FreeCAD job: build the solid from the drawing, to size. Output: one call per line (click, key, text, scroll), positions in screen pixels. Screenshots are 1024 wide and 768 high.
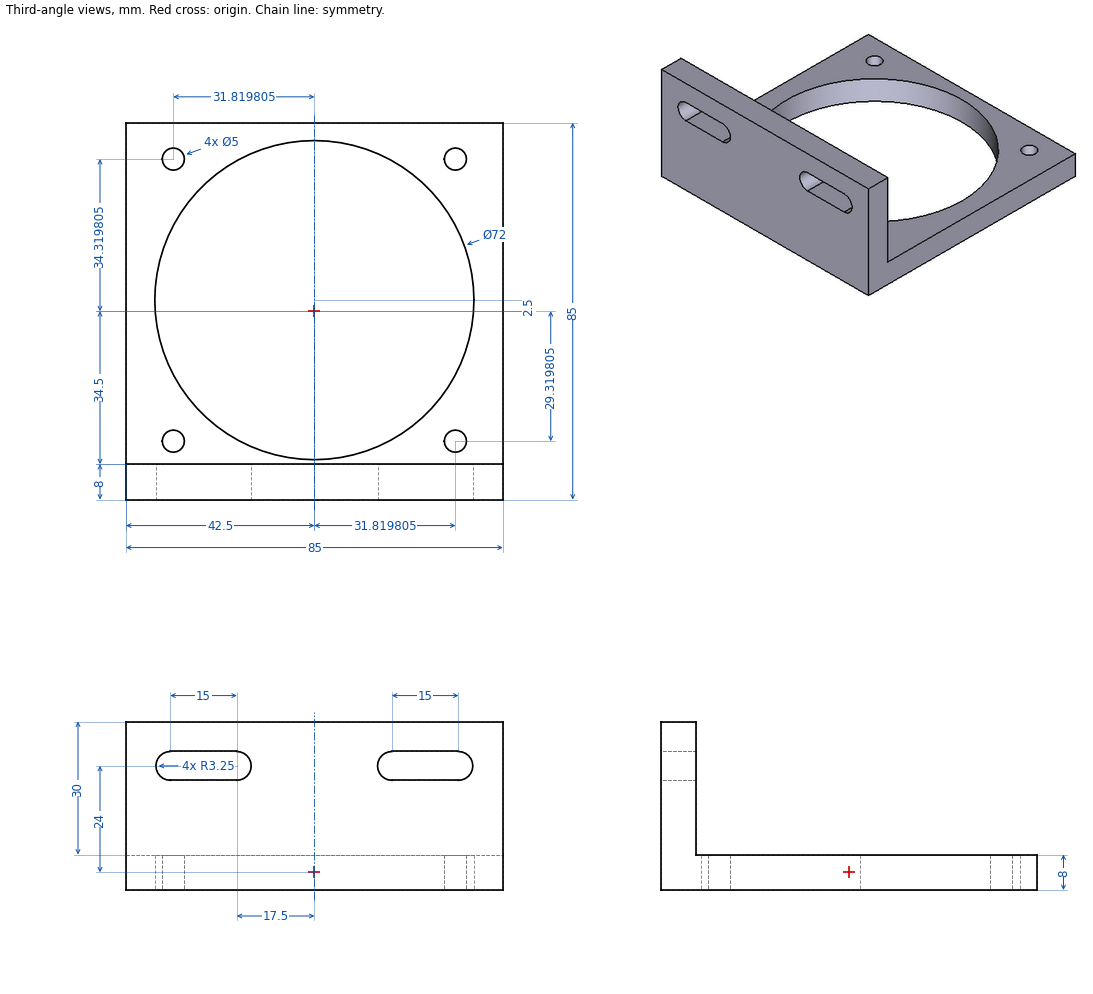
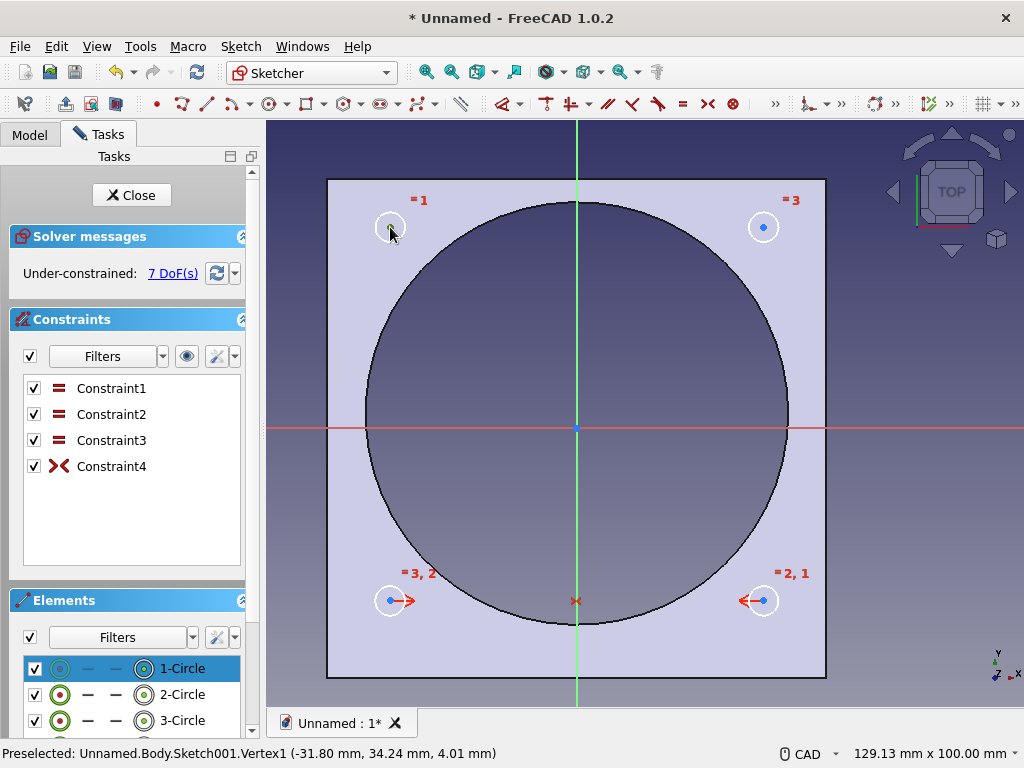
click(764, 227)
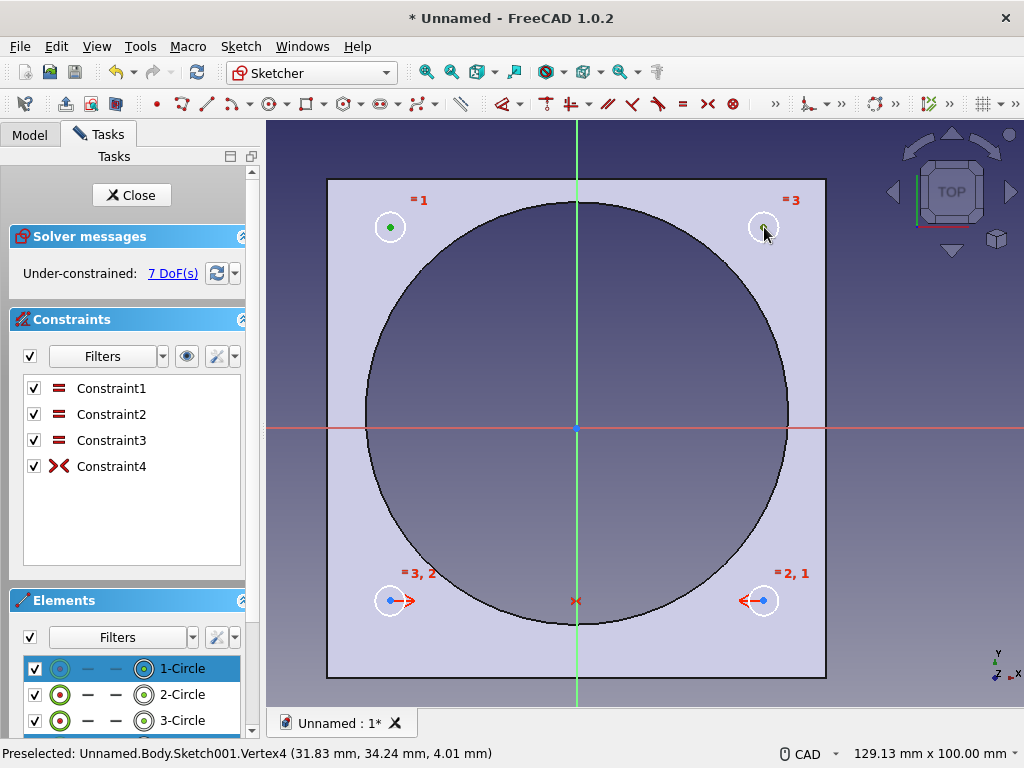
click(577, 641)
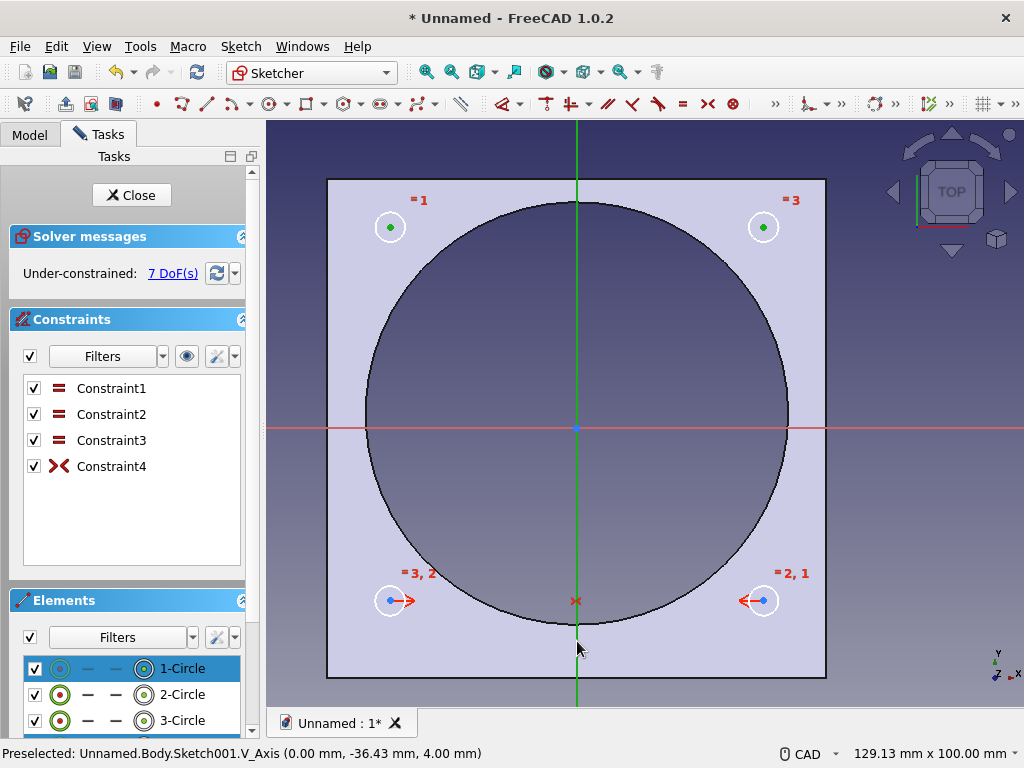
click(708, 104)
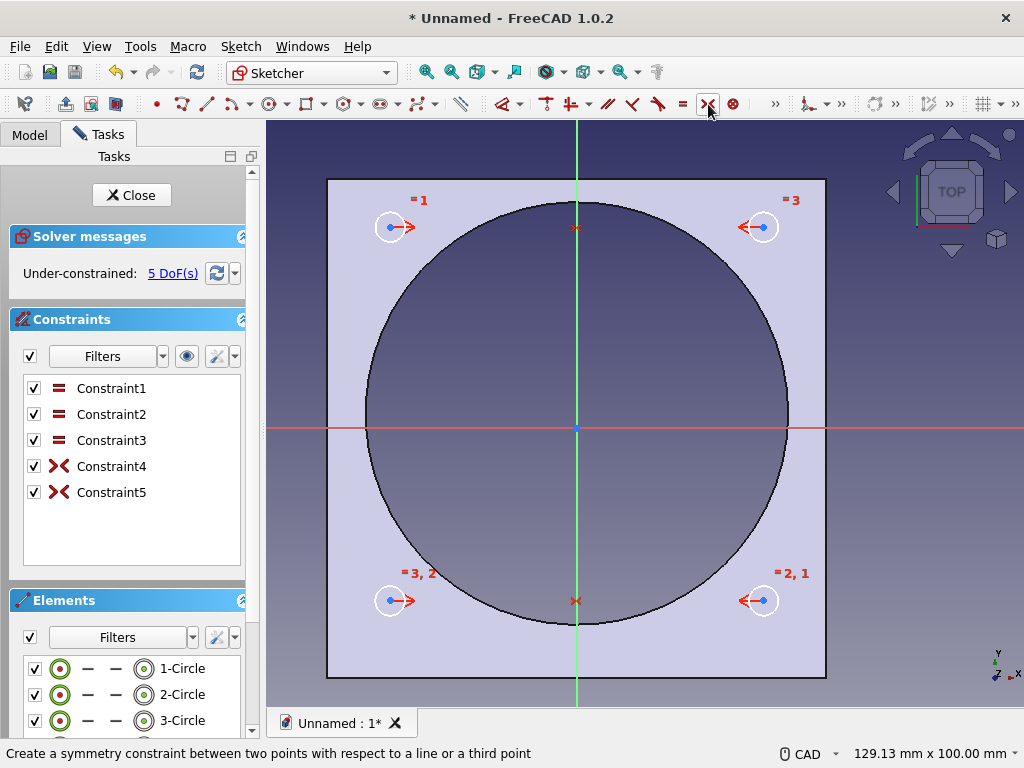
key(d)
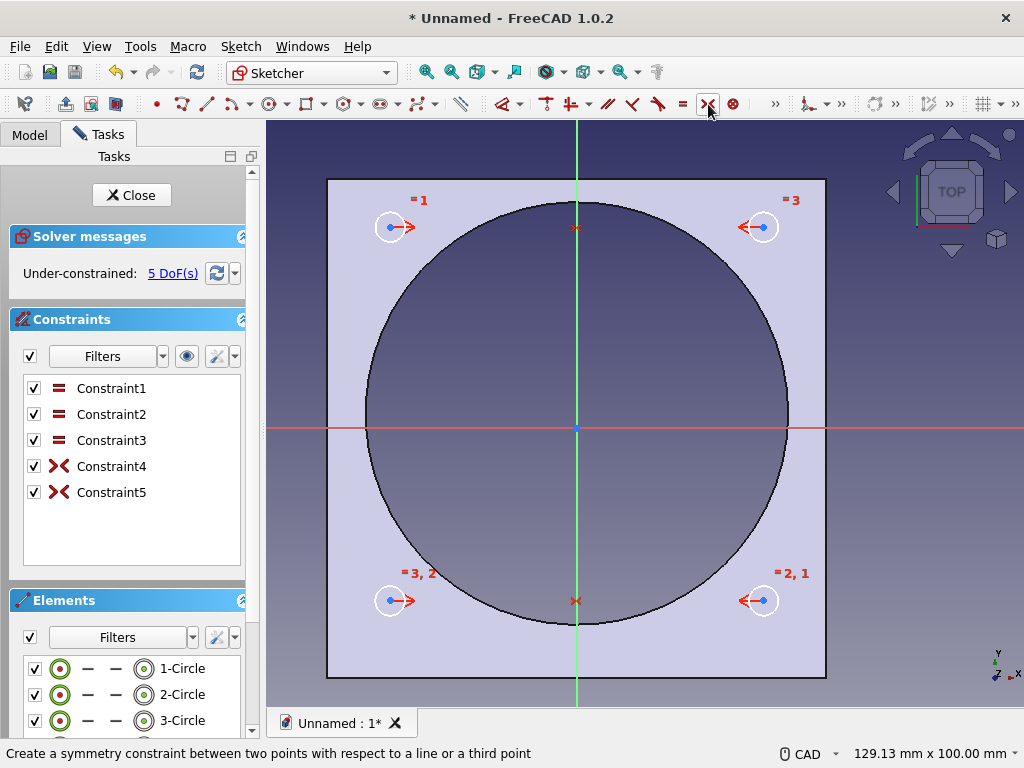
scroll(401, 217, up, 2)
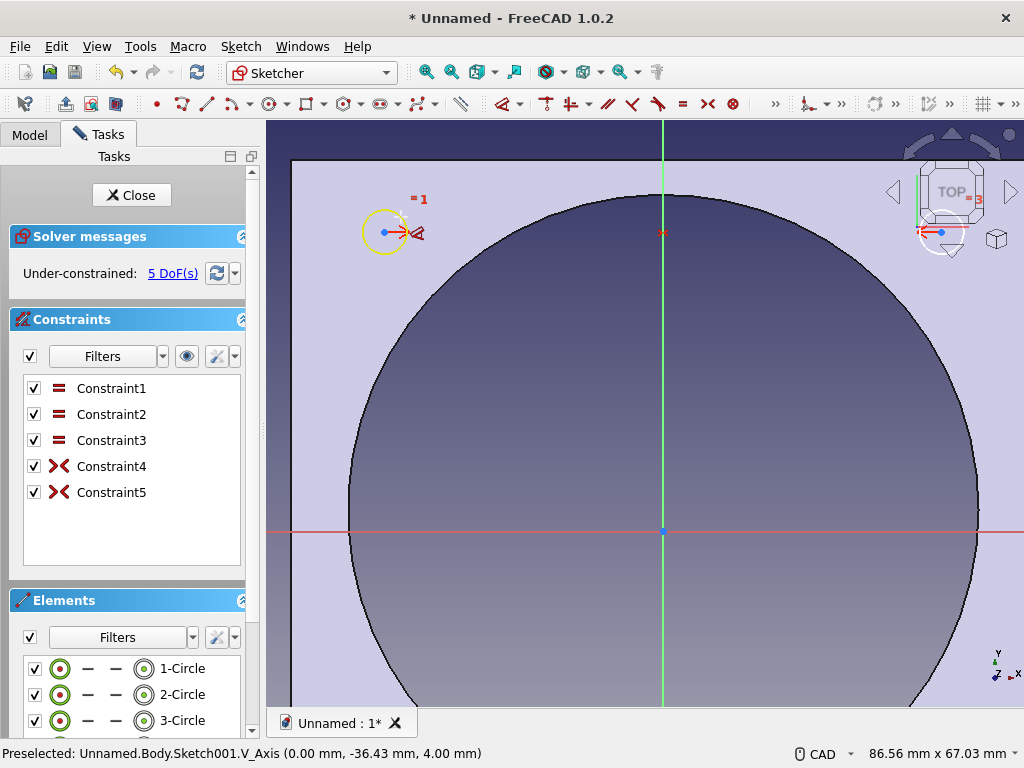
click(400, 217)
click(423, 194)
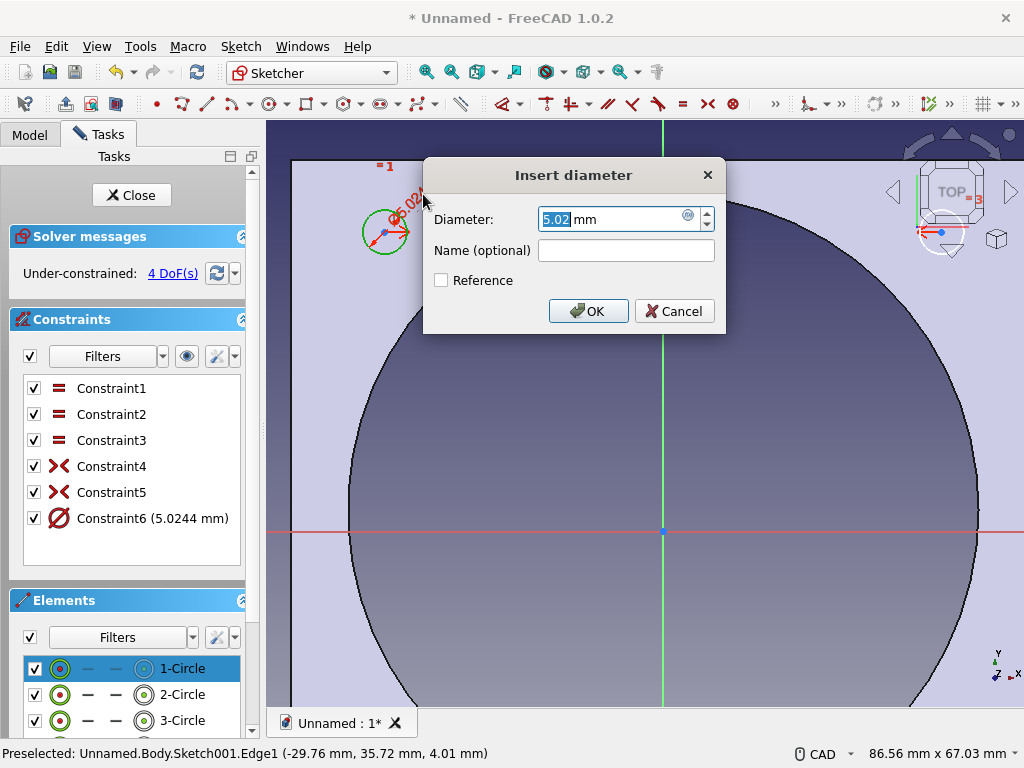
text(5)
key(Return)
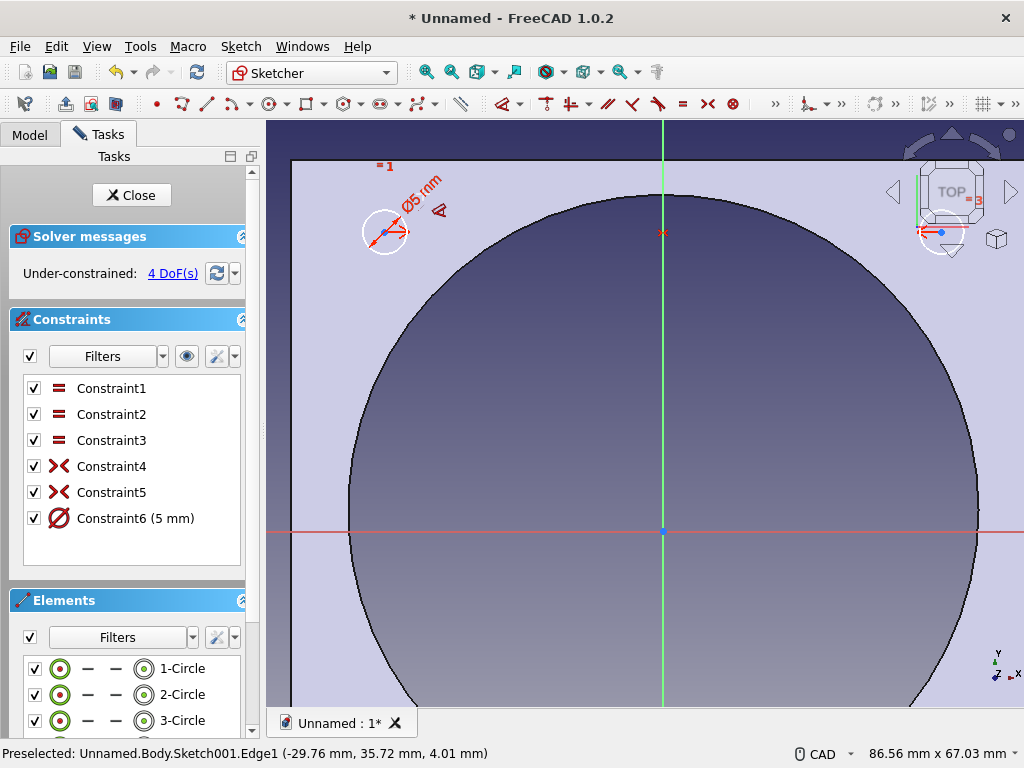
click(385, 232)
click(524, 198)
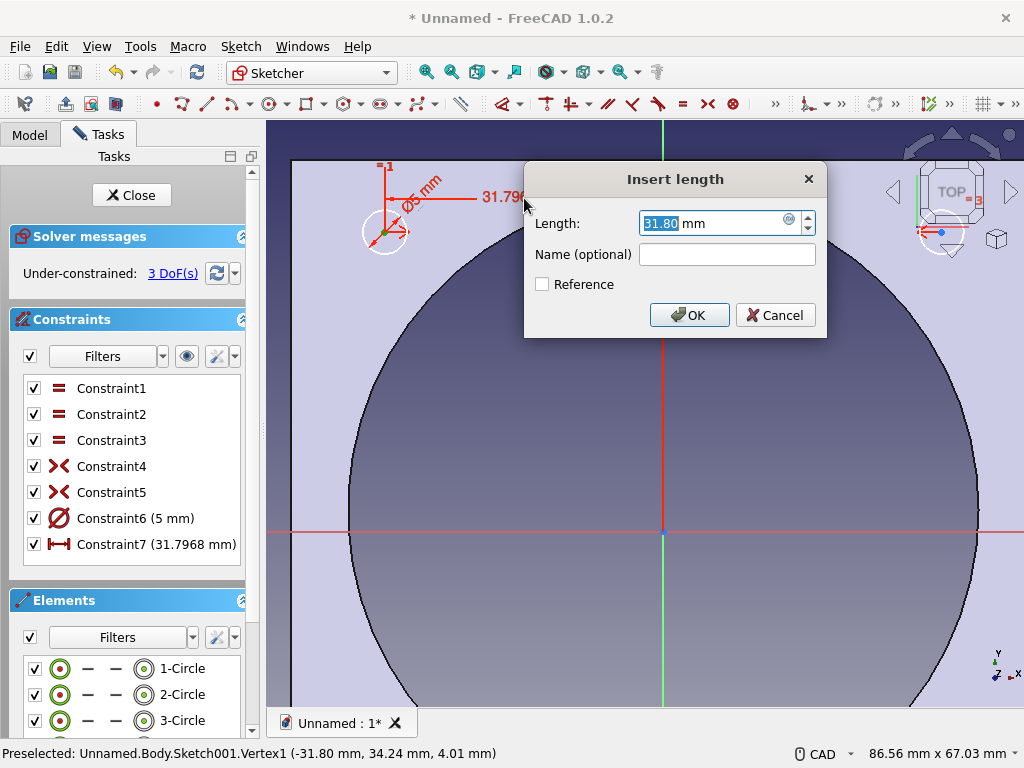
text(31.819805)
key(Return)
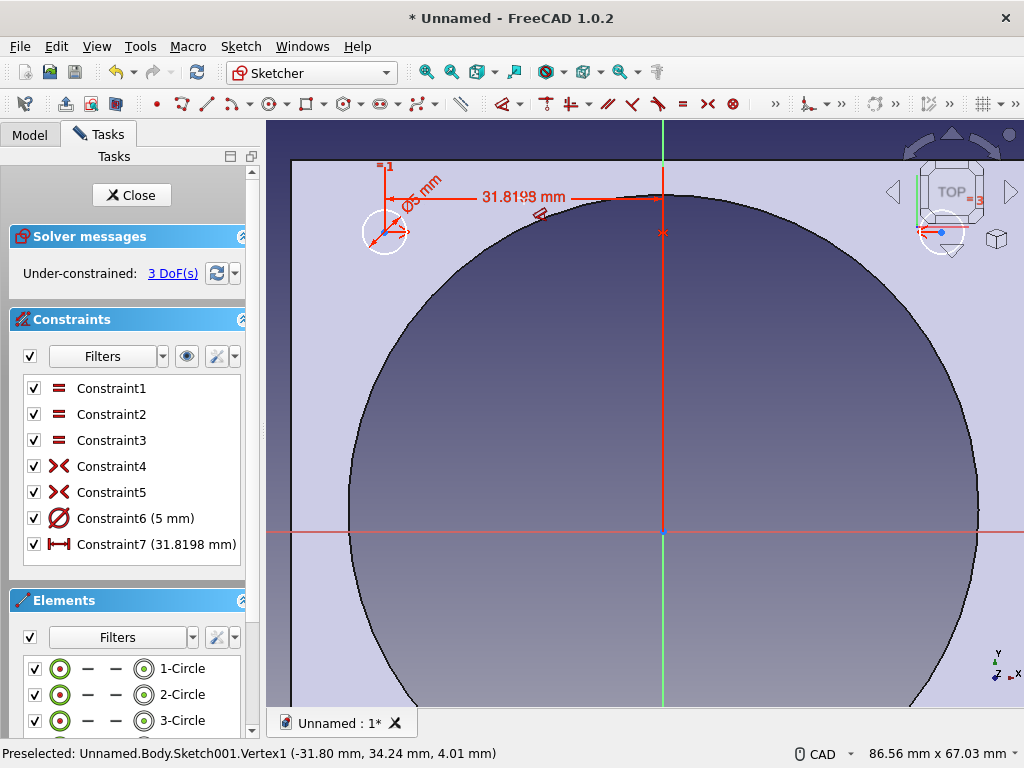
click(385, 232)
click(351, 382)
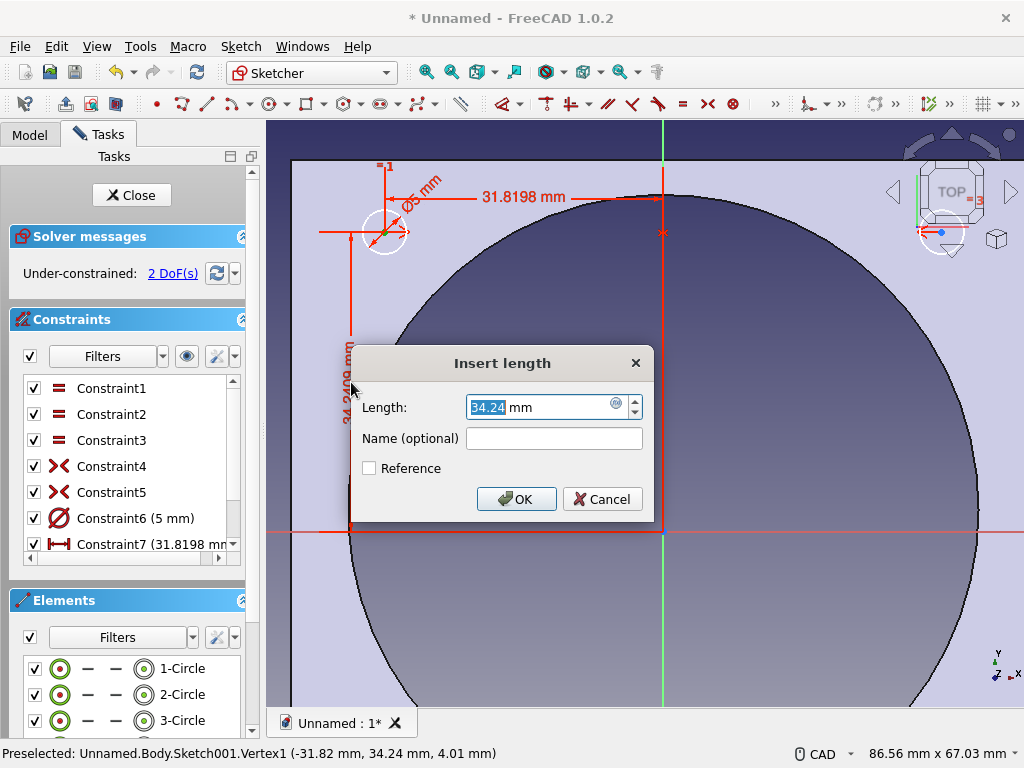
text(34.319805)
key(Return)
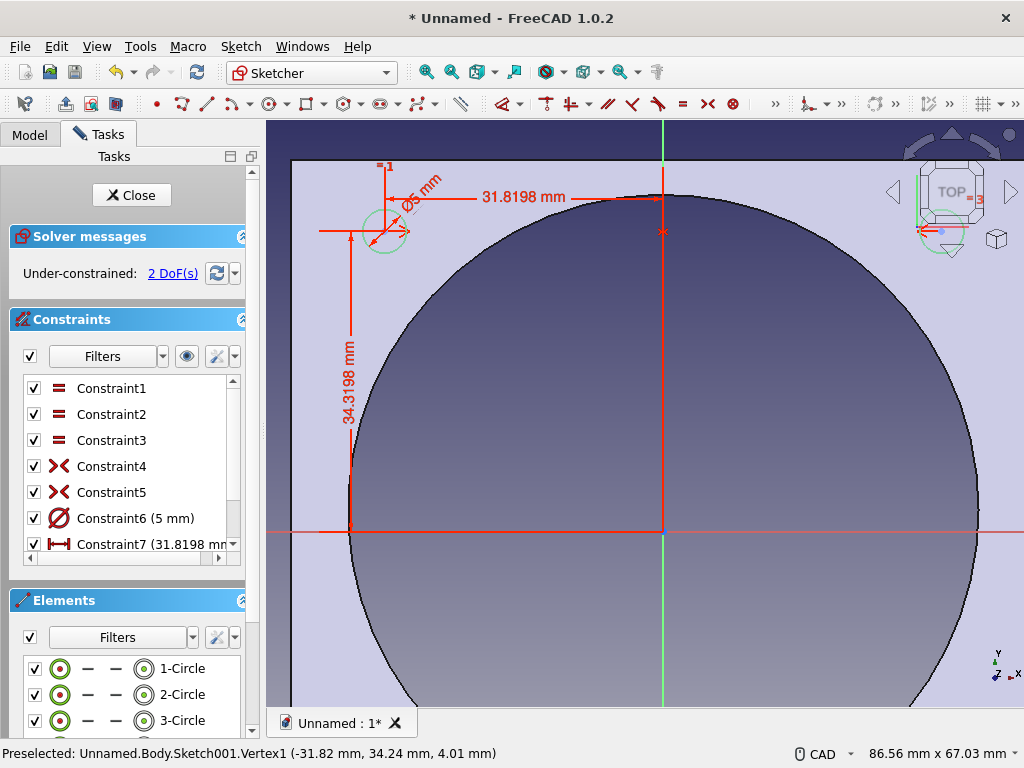
scroll(400, 217, down, 2)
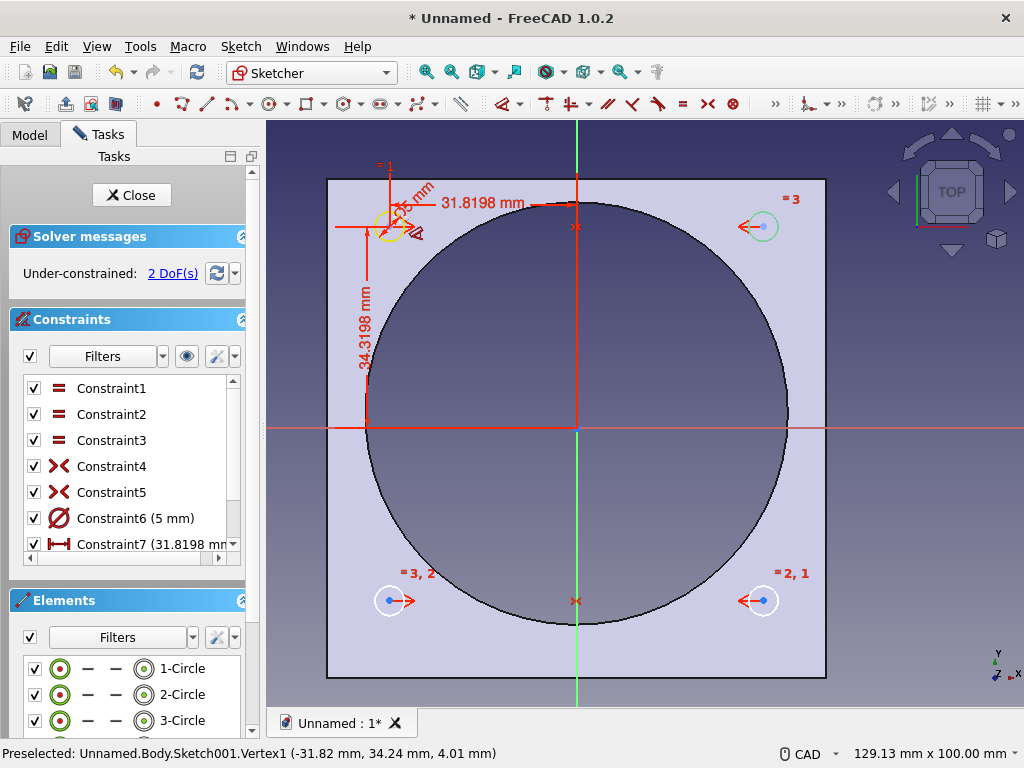
click(763, 601)
click(670, 635)